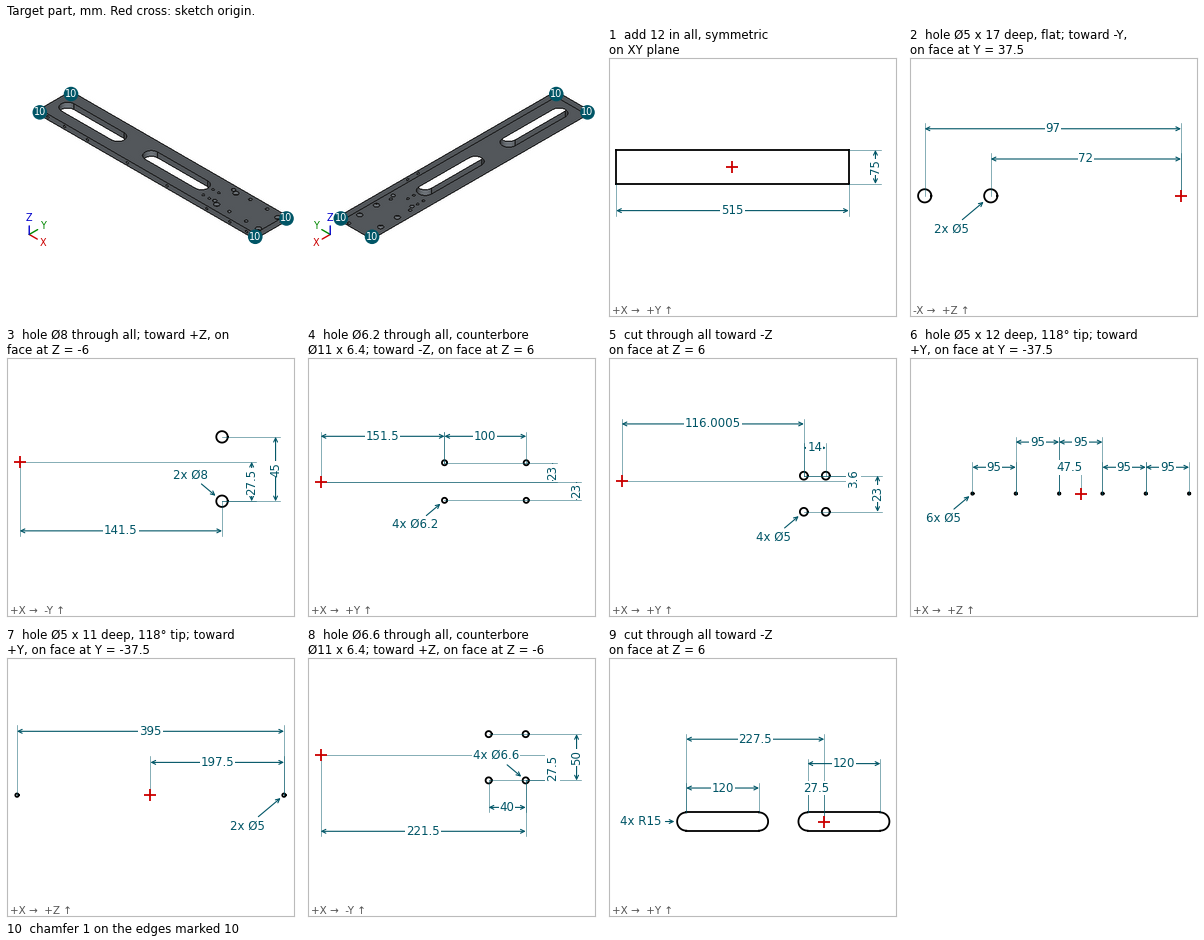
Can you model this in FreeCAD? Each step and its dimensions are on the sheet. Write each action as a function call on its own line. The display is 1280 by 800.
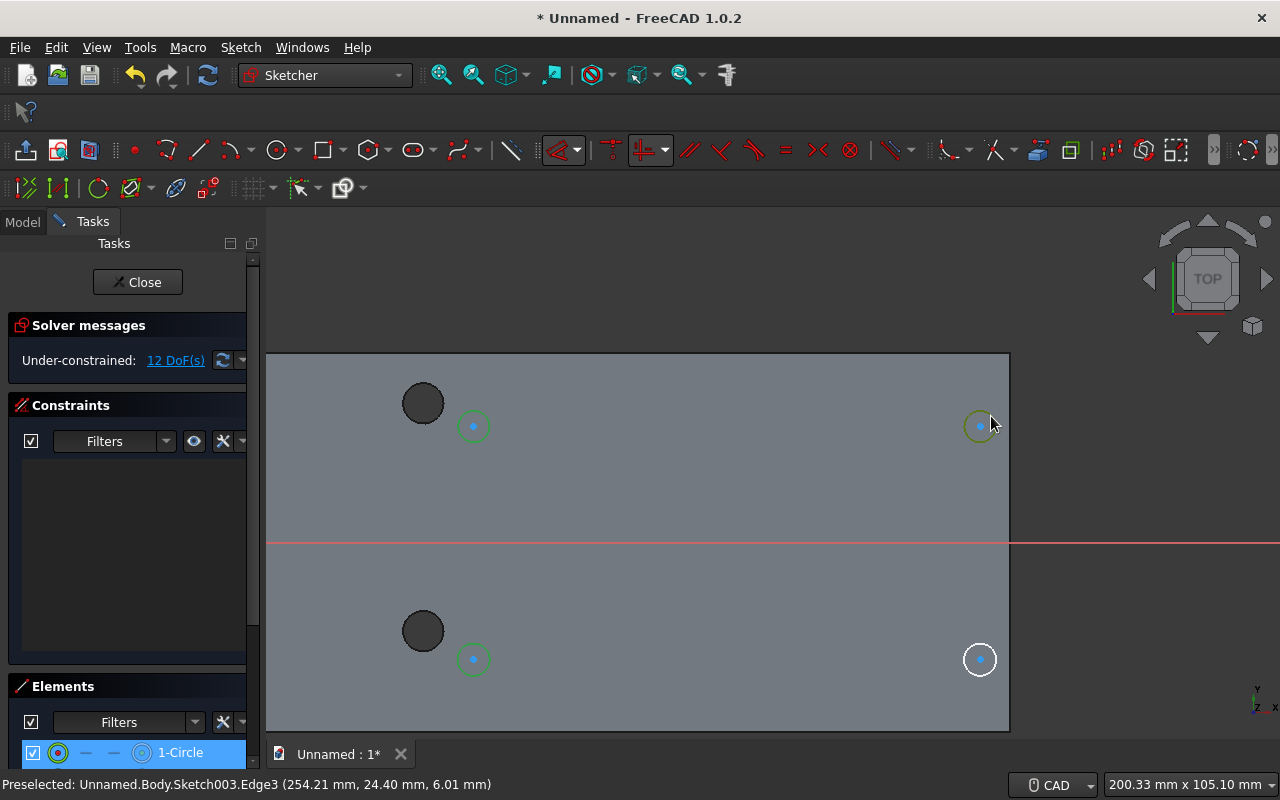
click(991, 648)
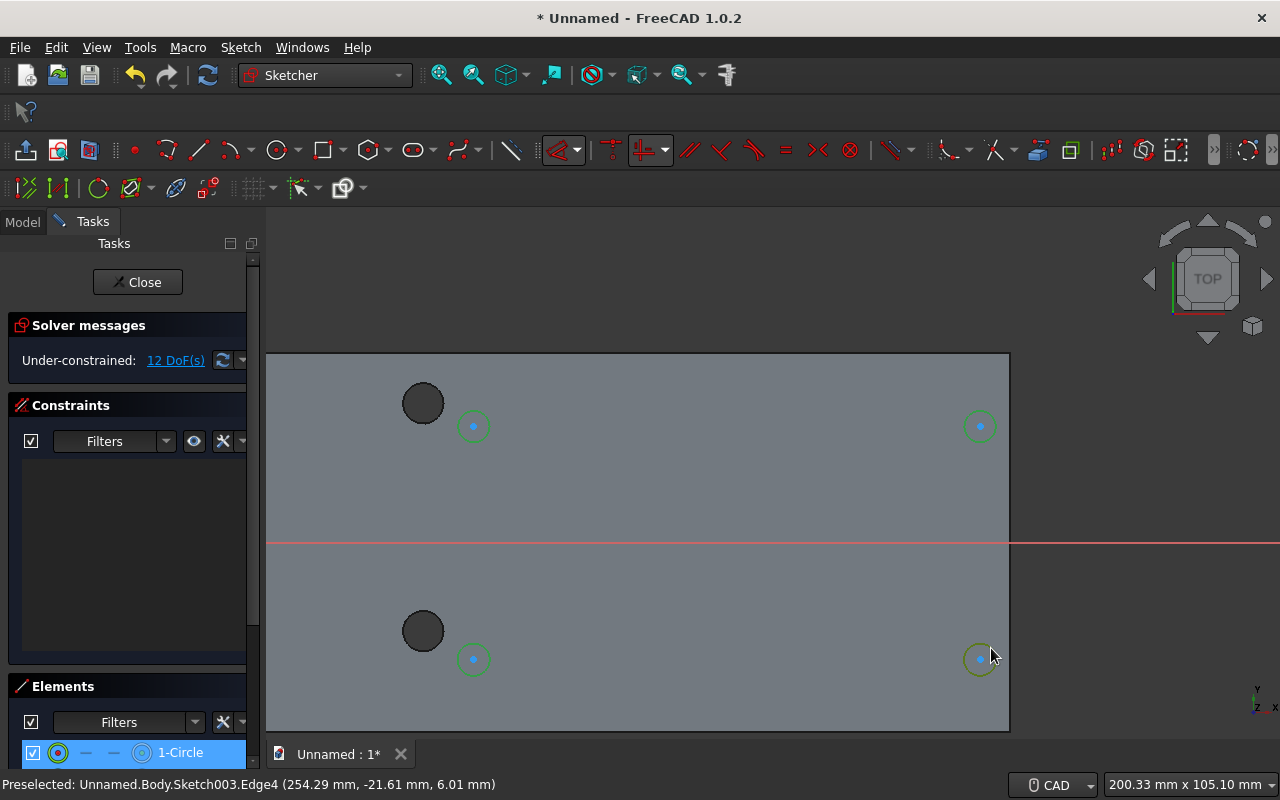
click(786, 150)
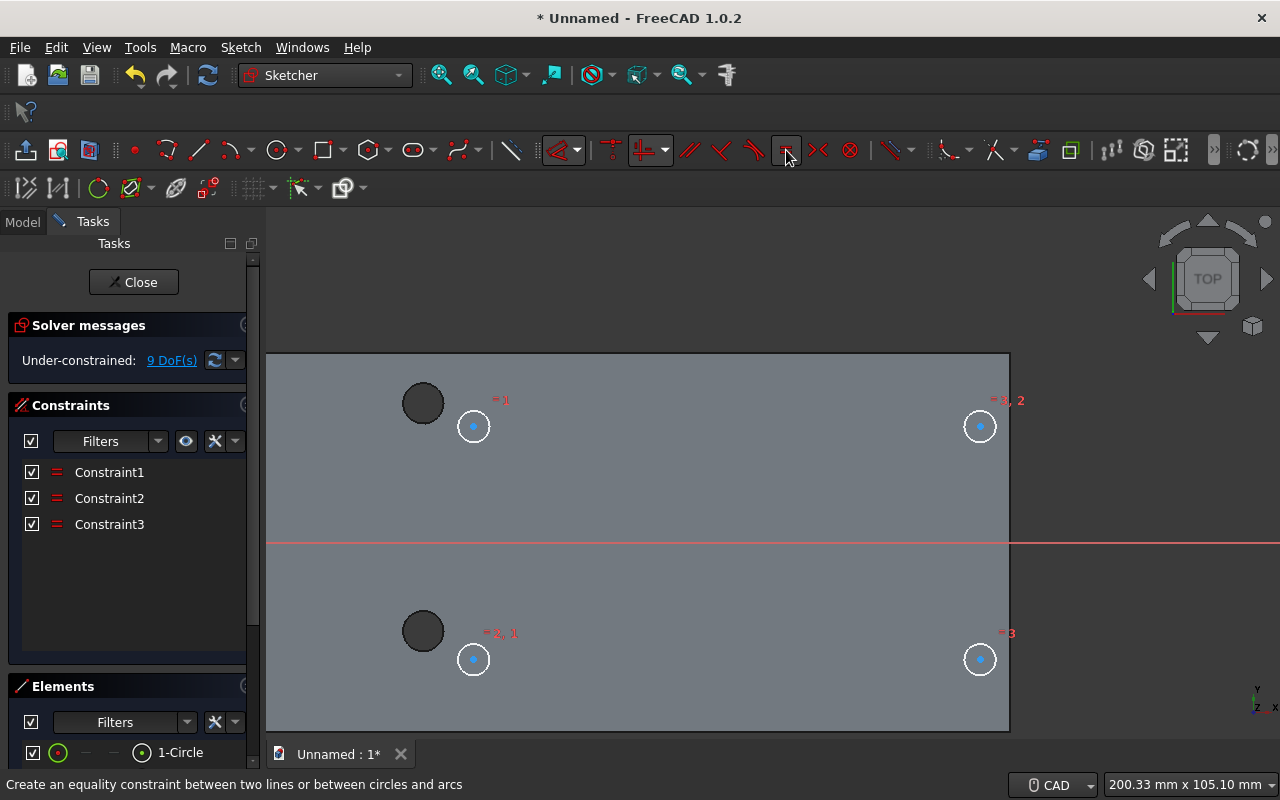
click(474, 427)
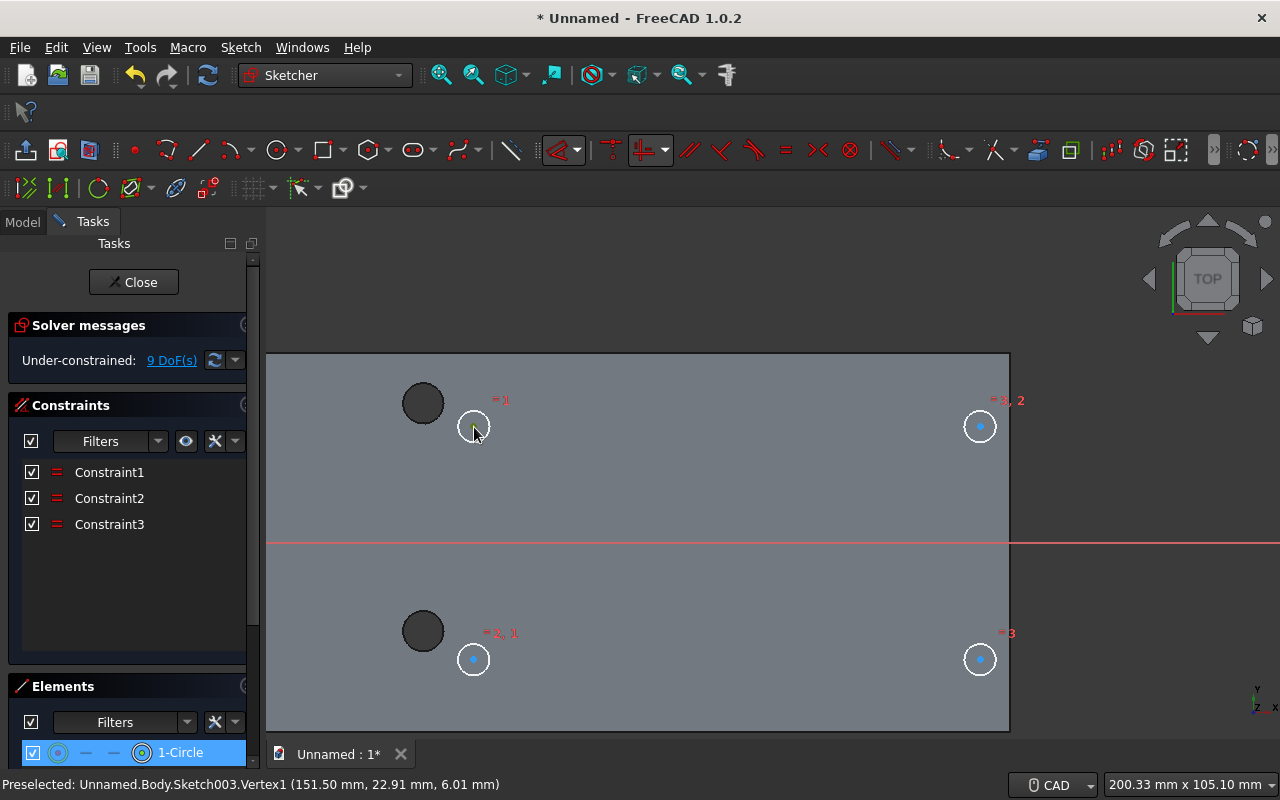
click(474, 660)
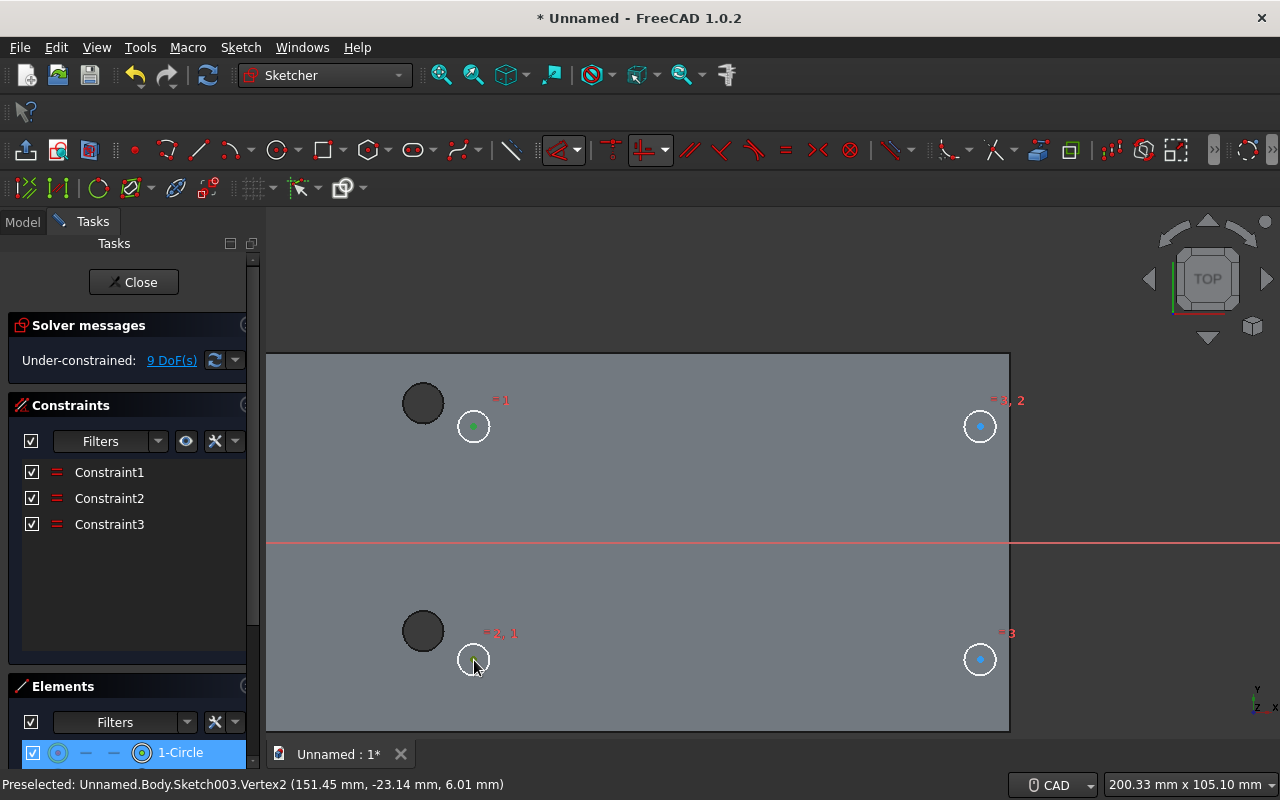
key(v)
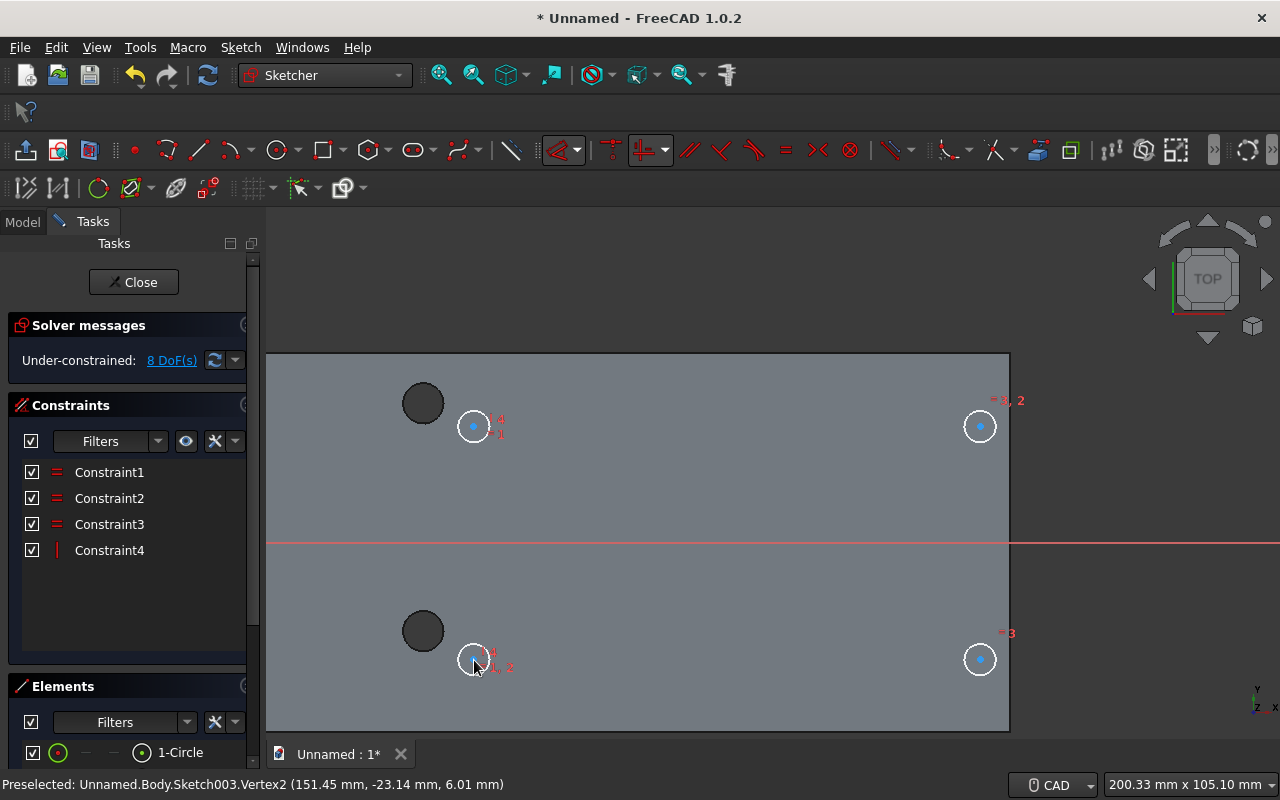
click(474, 427)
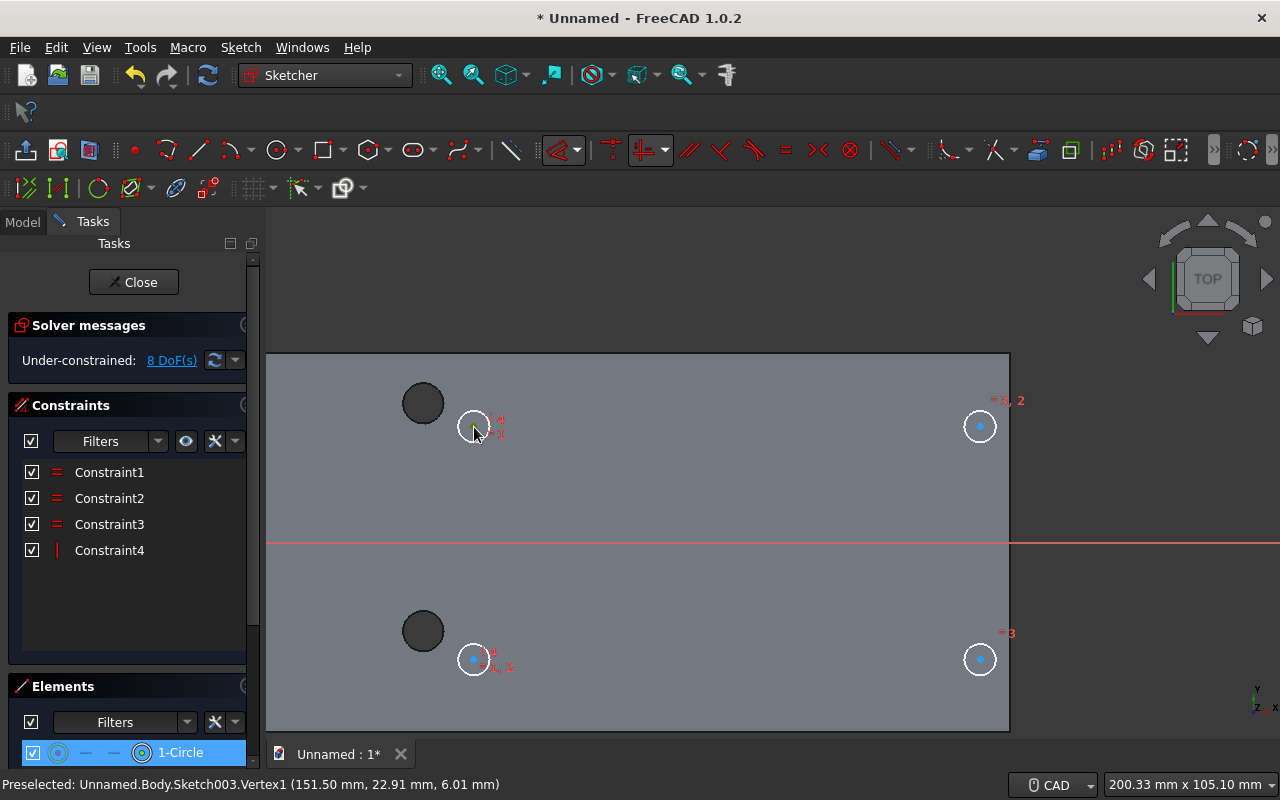
click(980, 427)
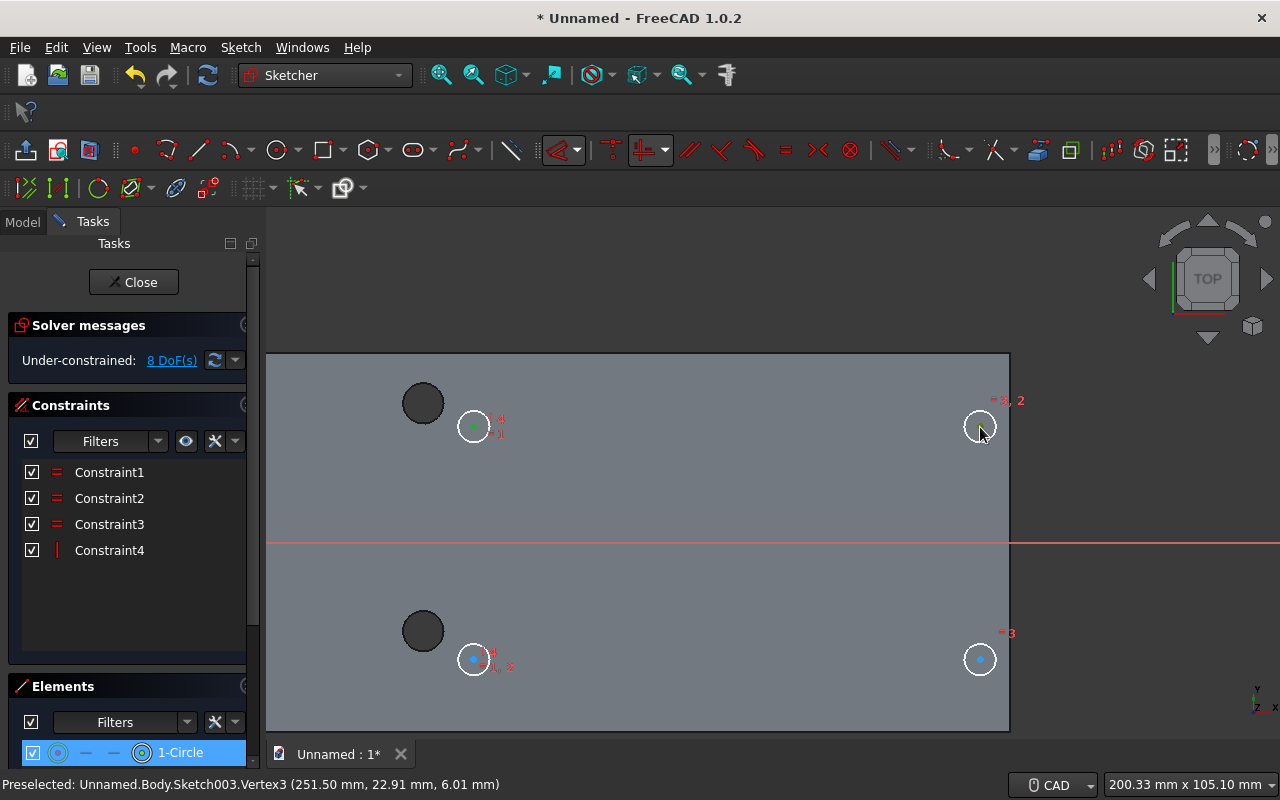
key(h)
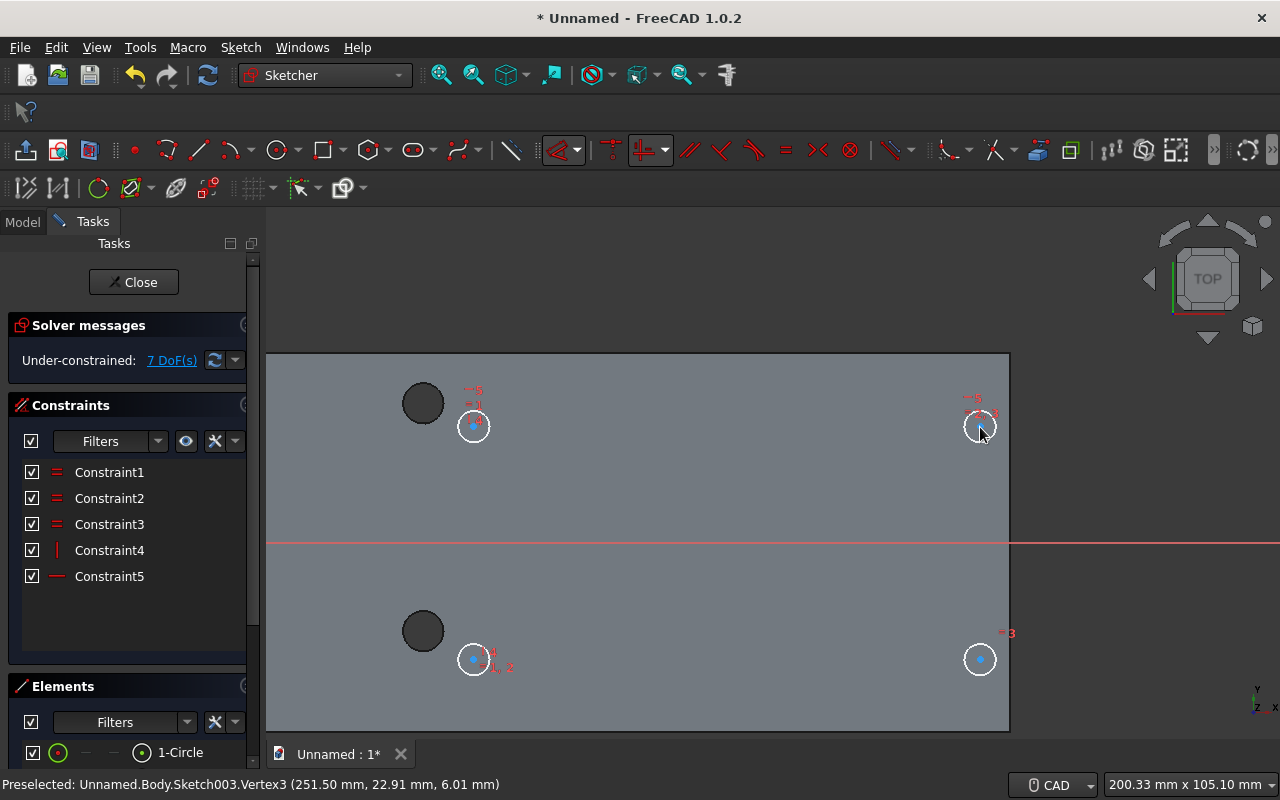
click(980, 427)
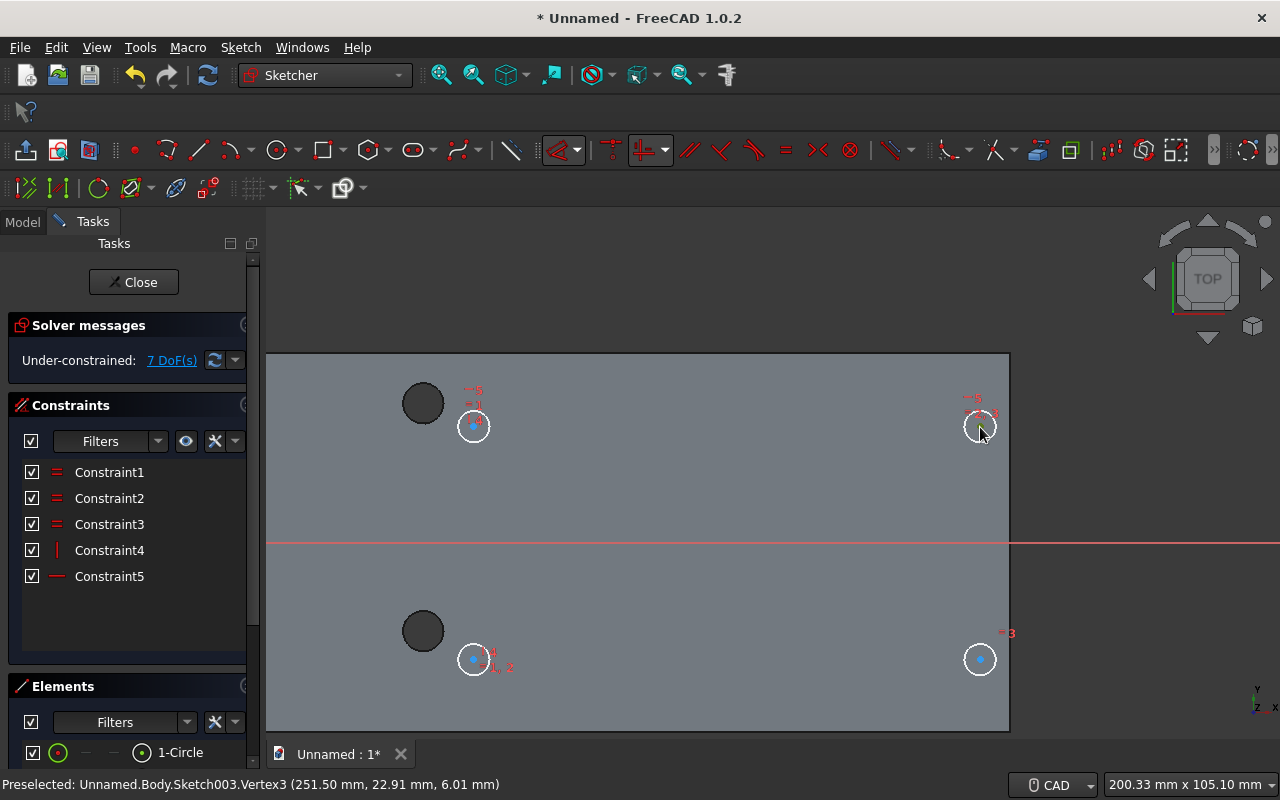
click(980, 660)